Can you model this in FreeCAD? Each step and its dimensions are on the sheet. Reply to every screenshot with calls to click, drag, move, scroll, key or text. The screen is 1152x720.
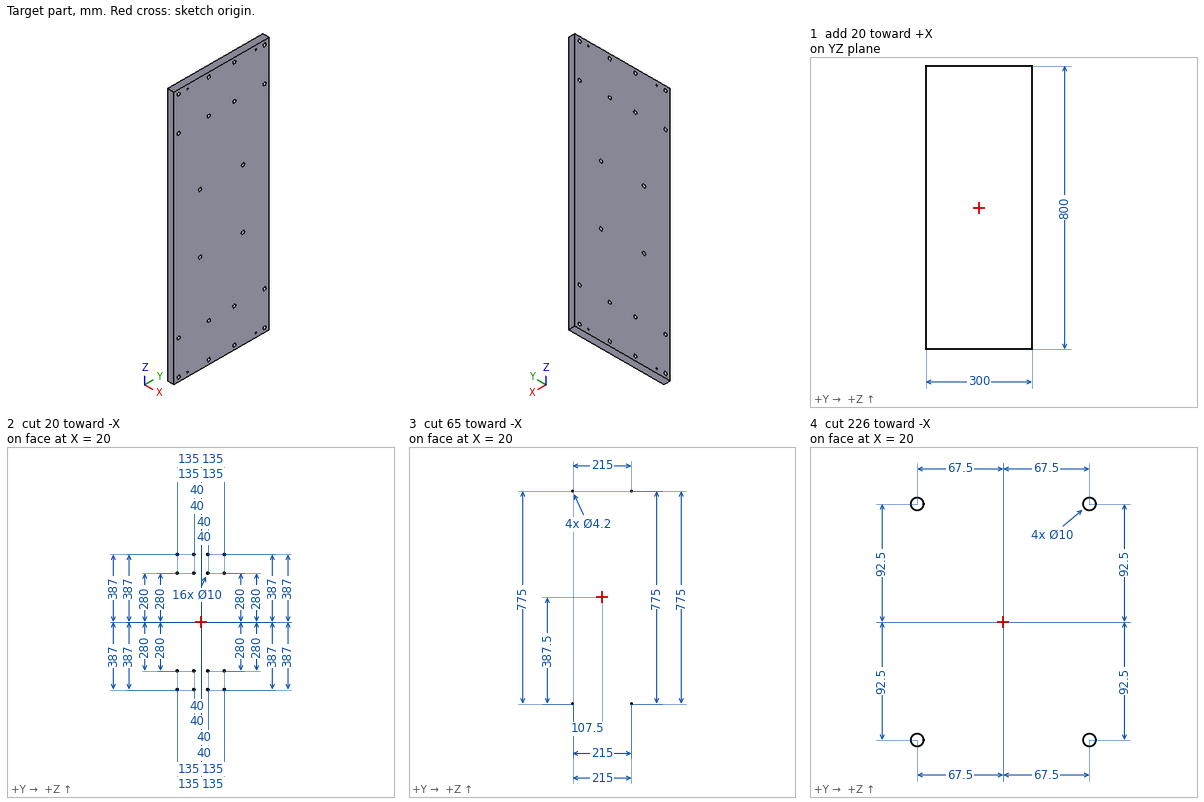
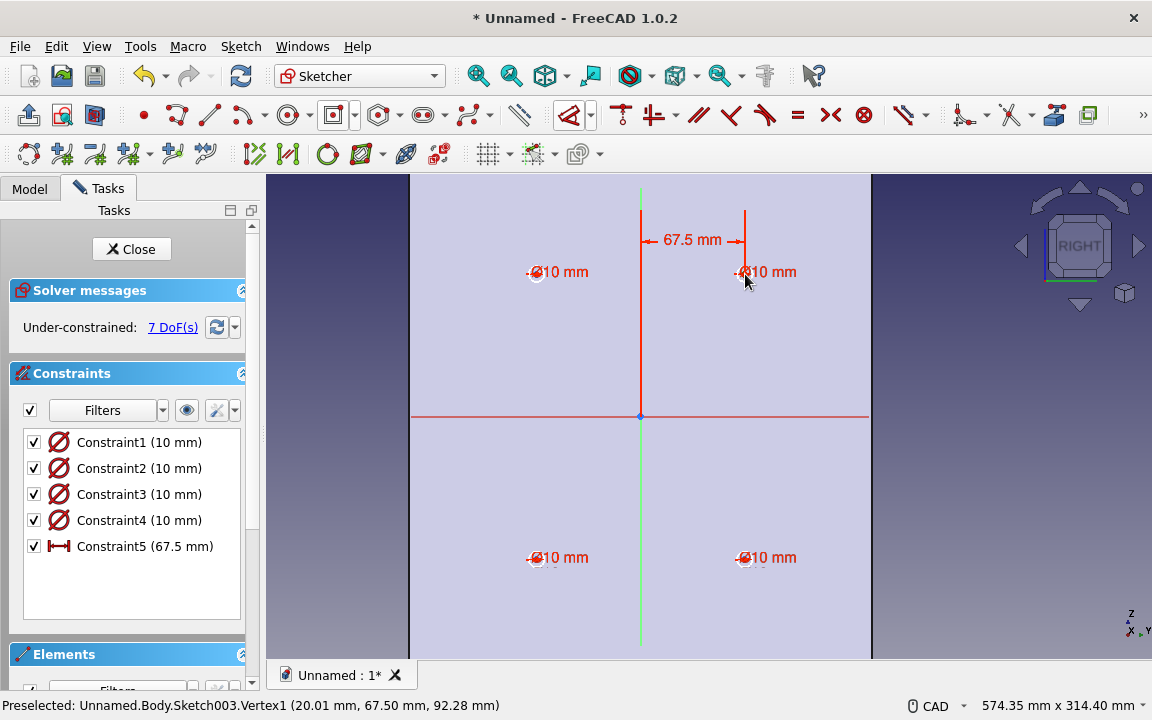
click(590, 116)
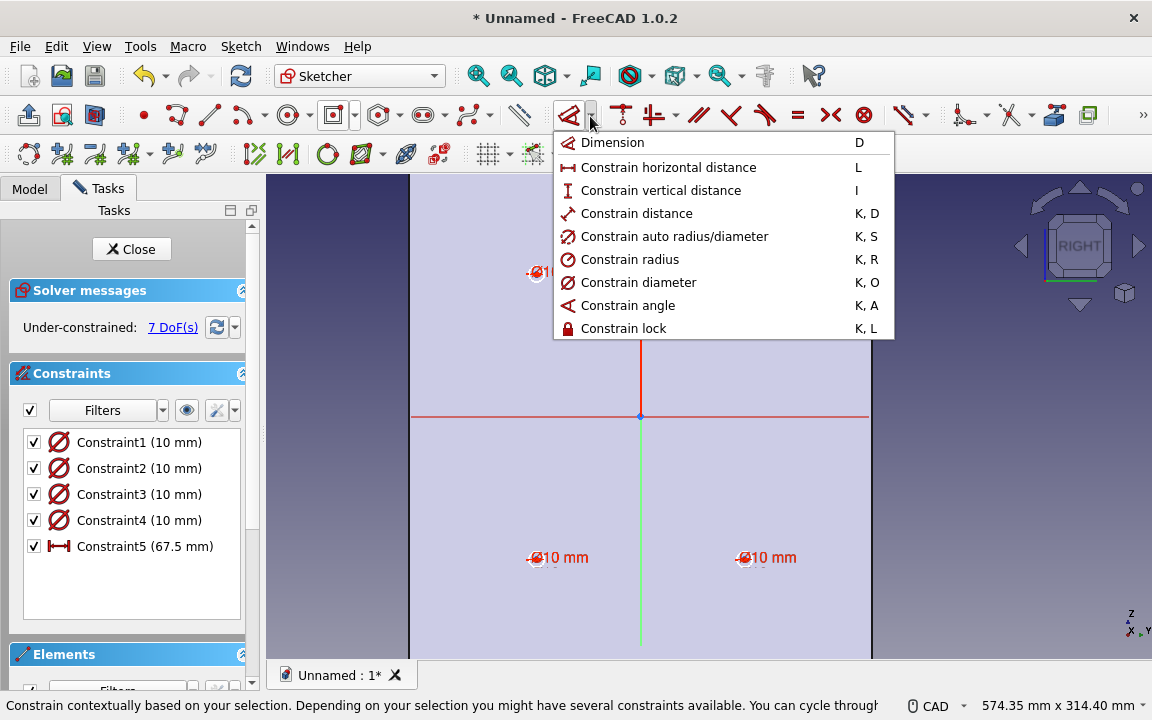
click(724, 190)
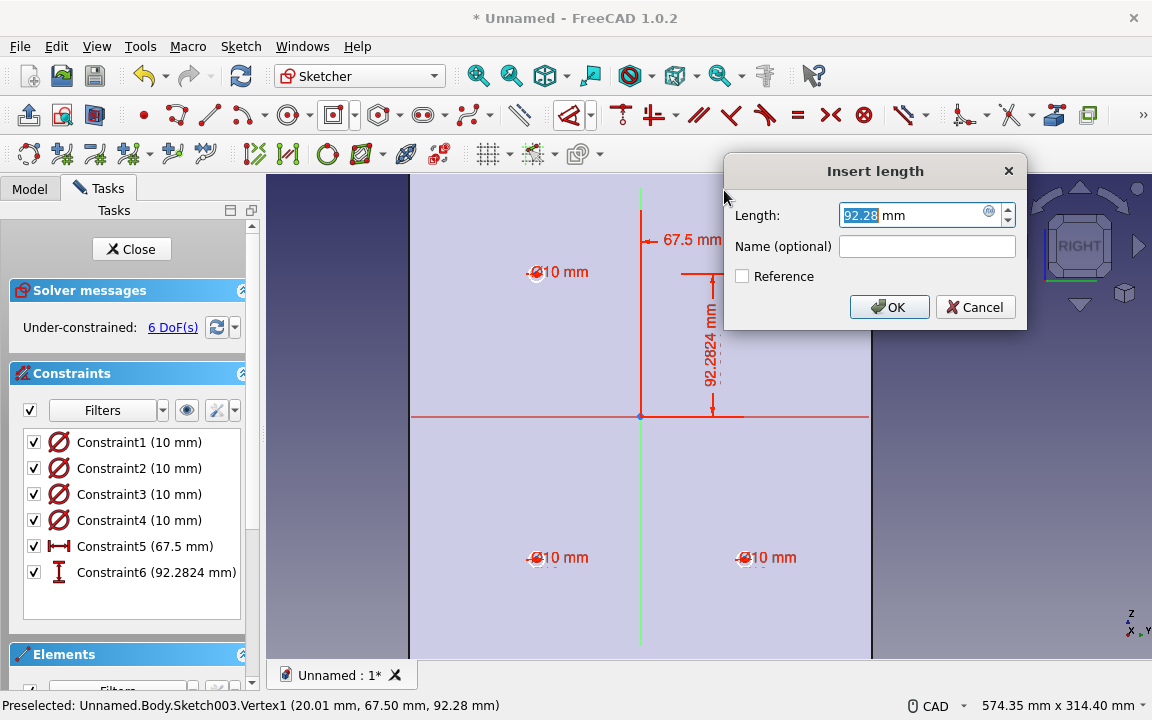
text(92.5)
key(Return)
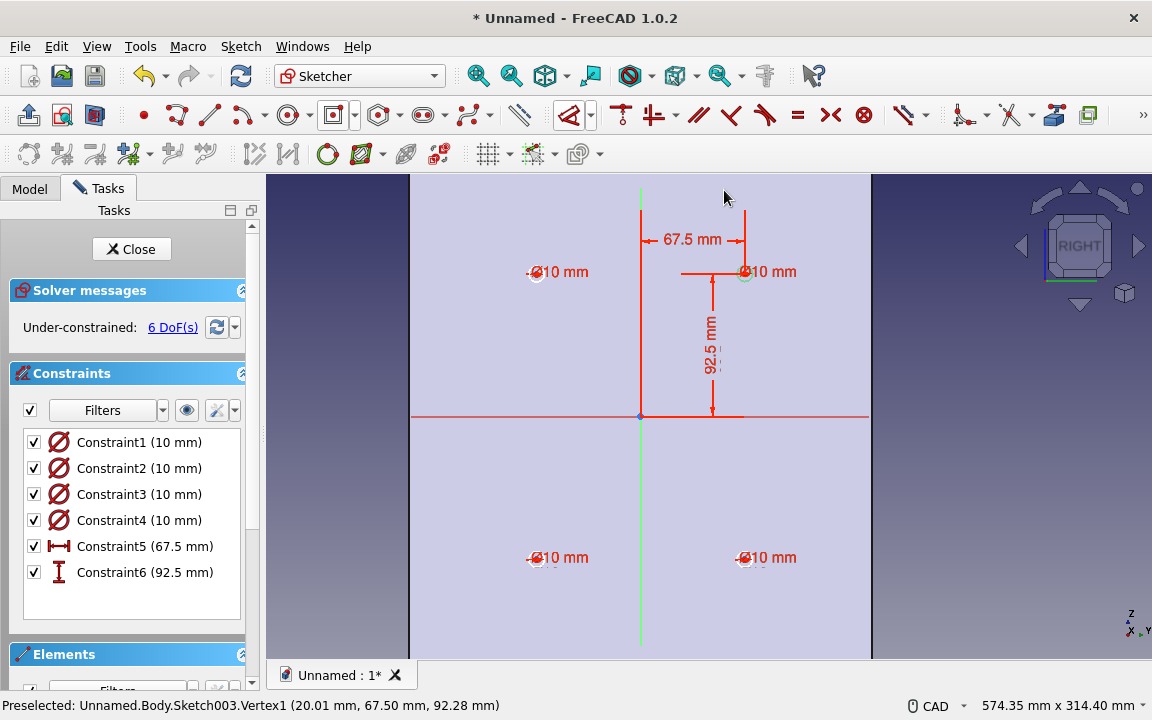
click(745, 560)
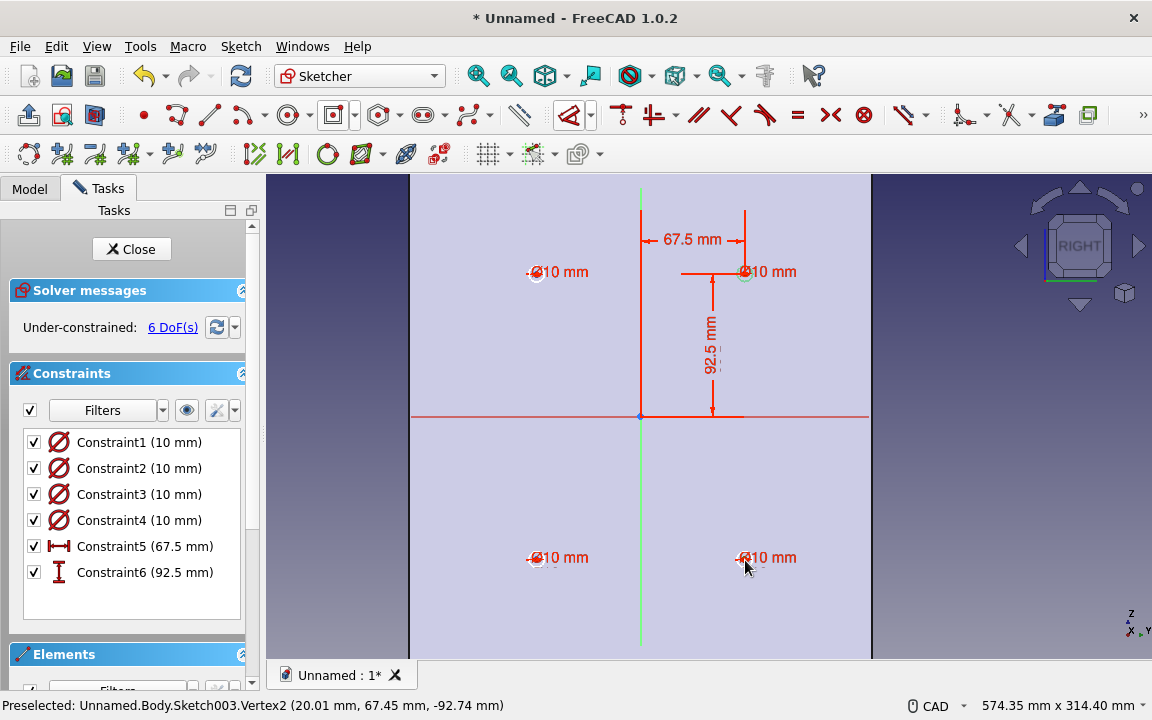
key(l)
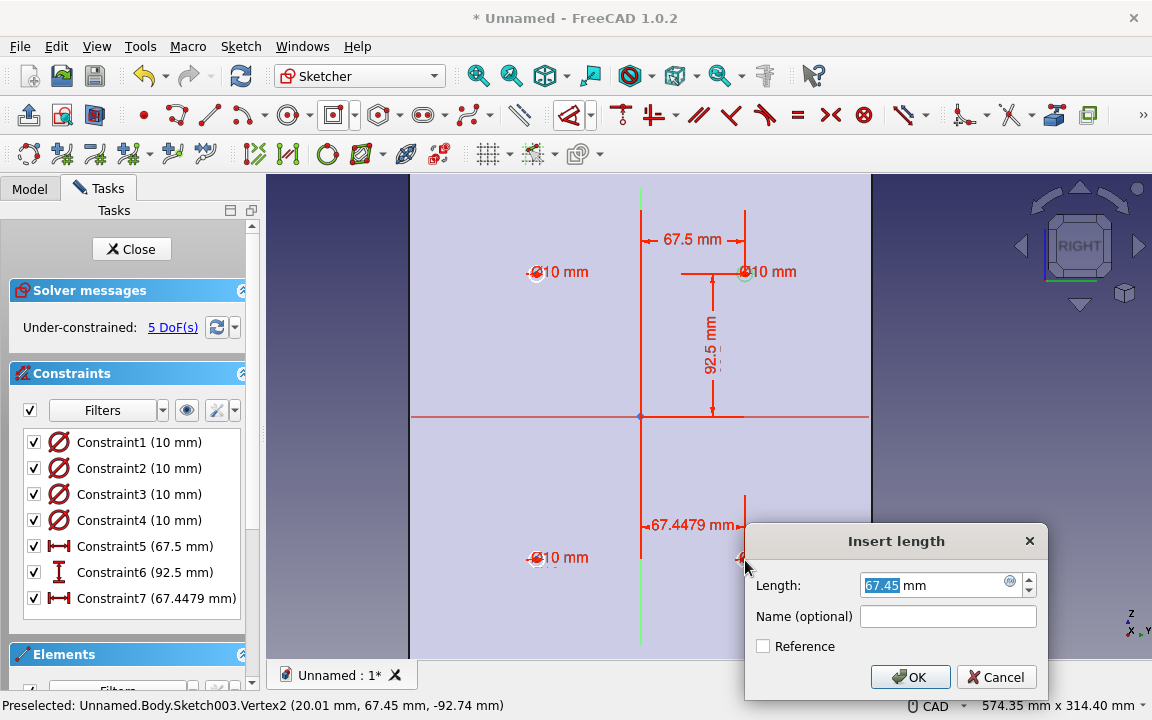
text(67.5)
key(Return)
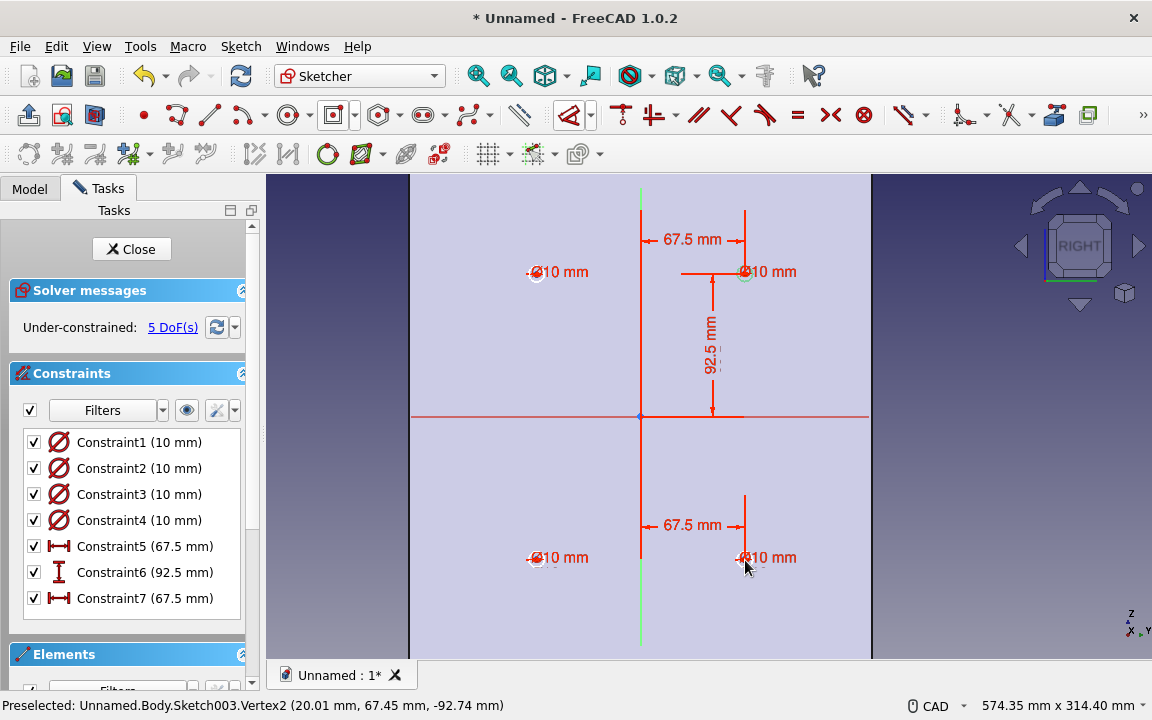
click(745, 560)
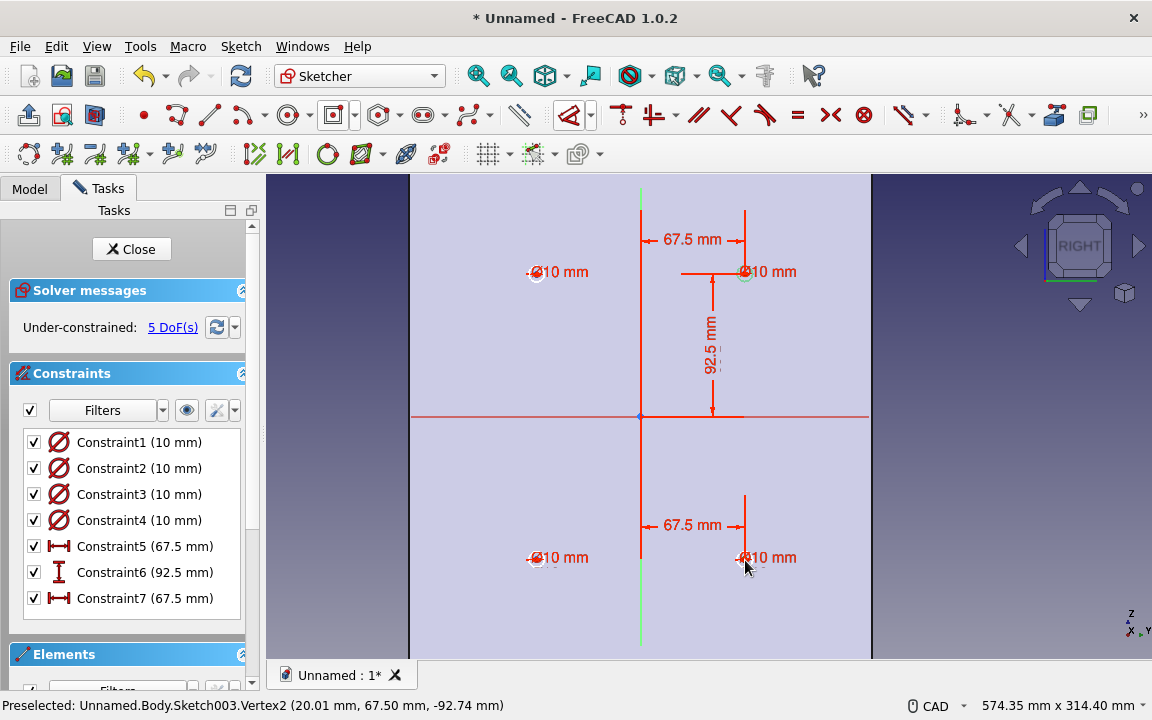
key(i)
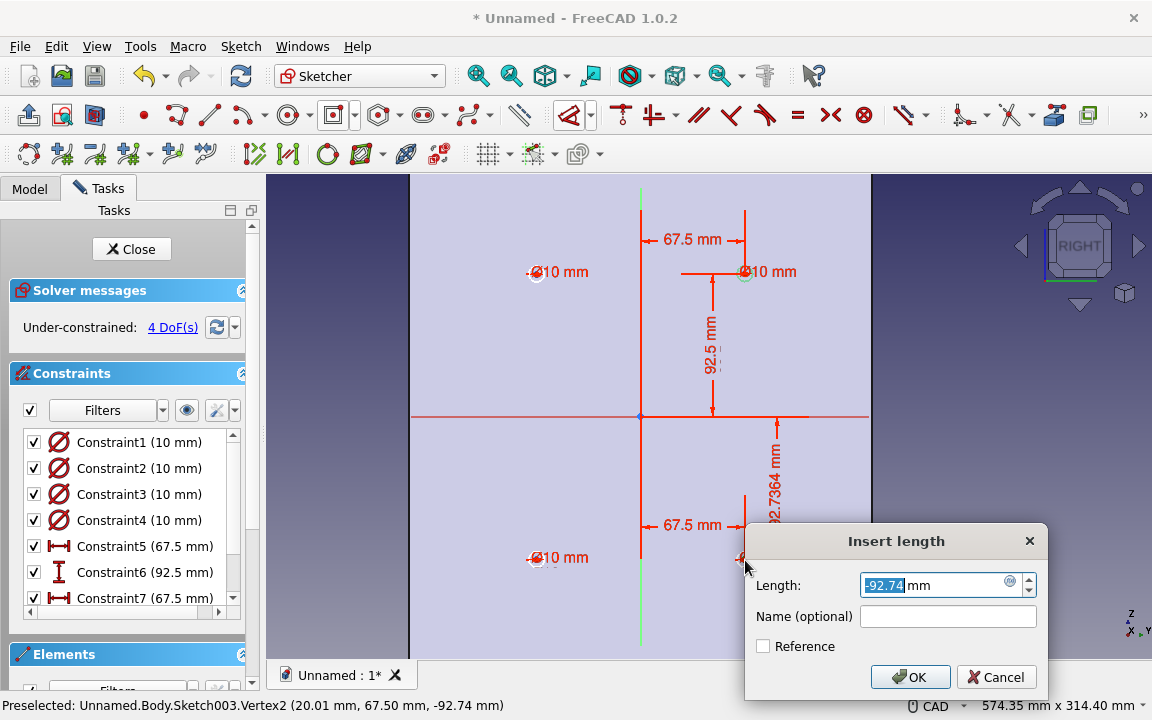
text(-92.5)
key(Return)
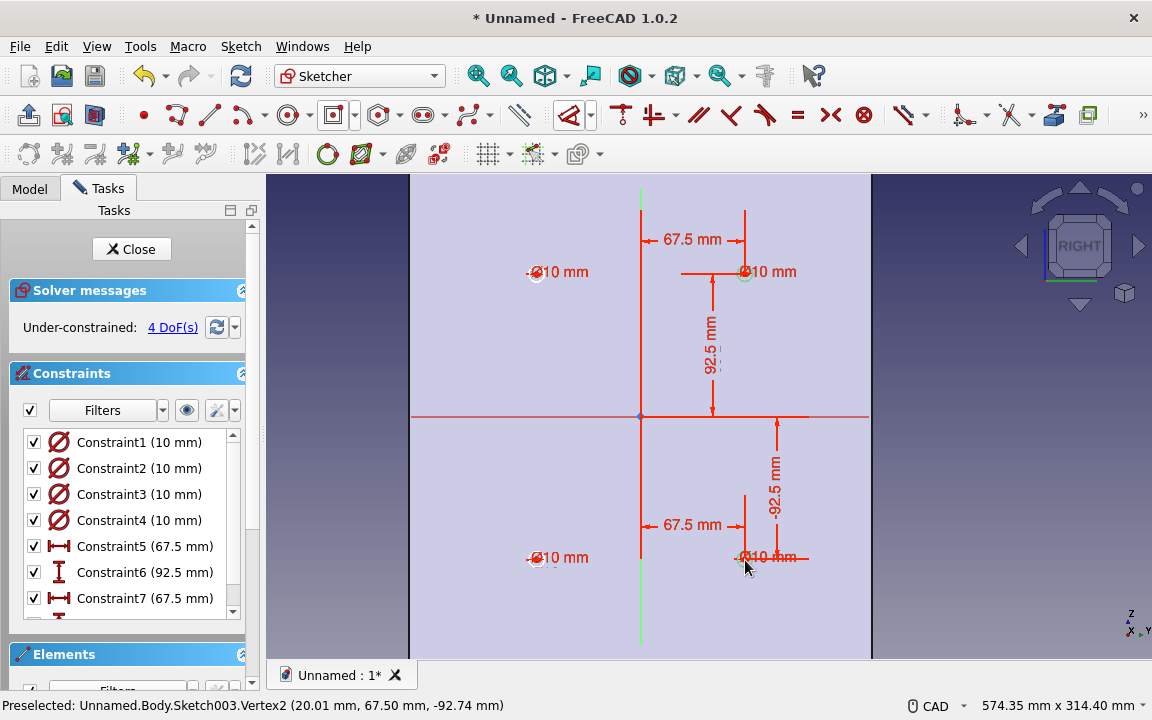
click(537, 560)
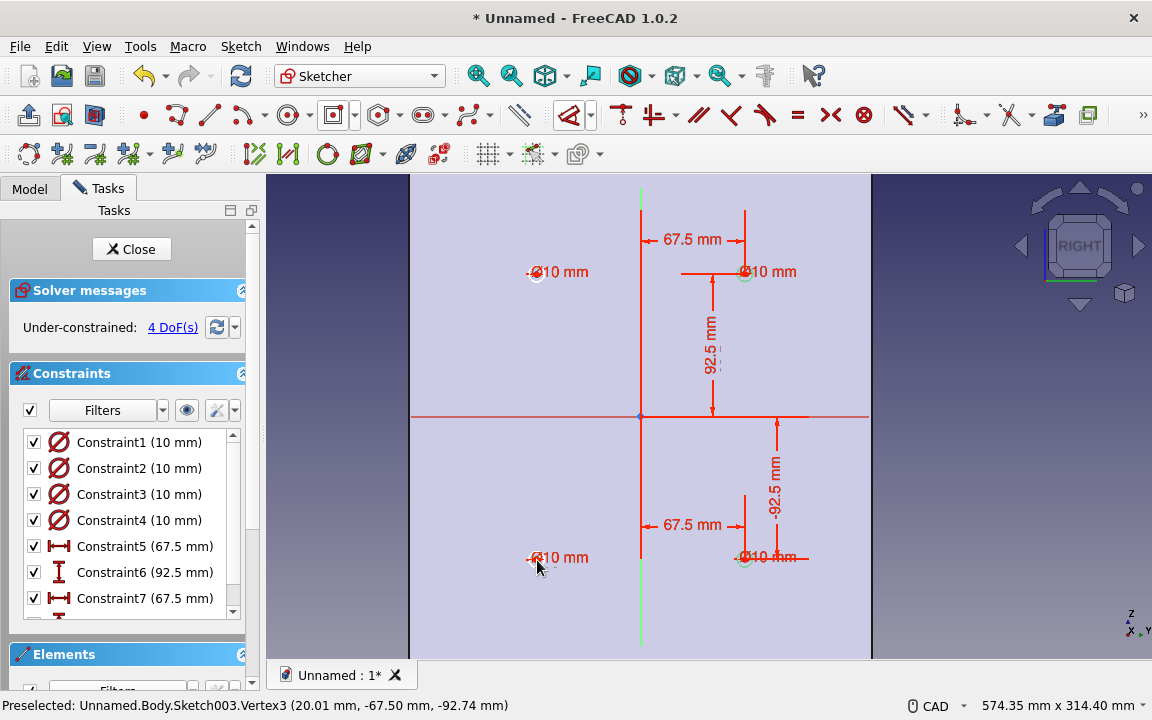
key(l)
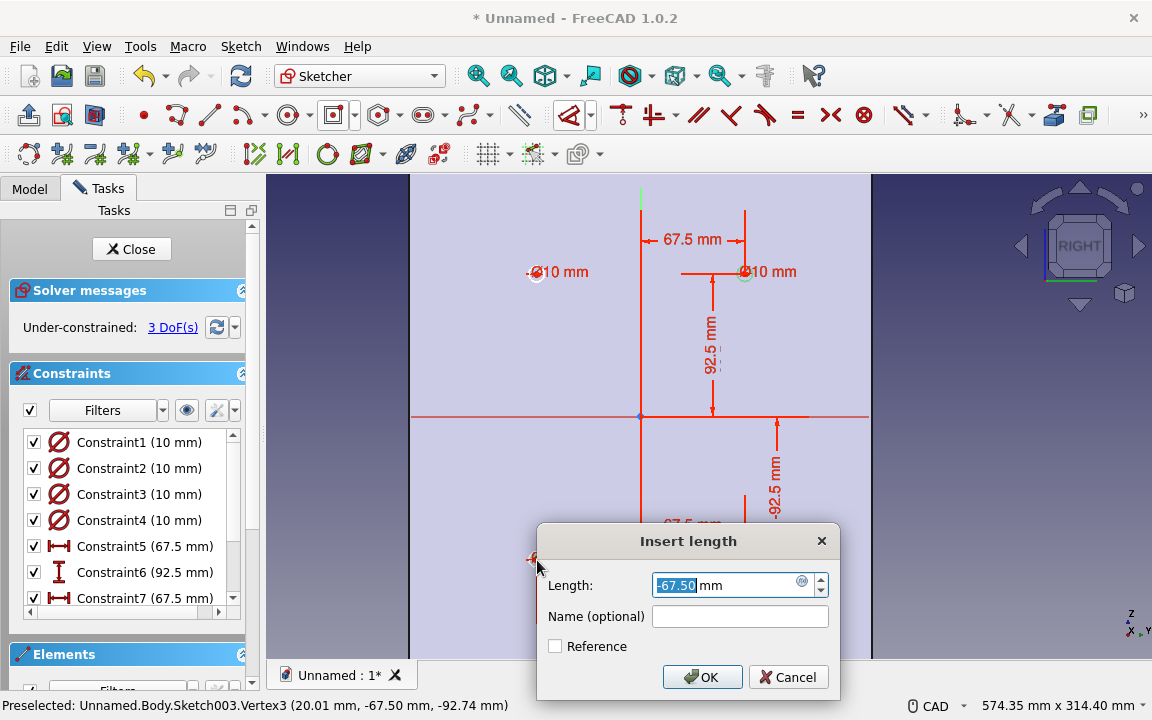
text(-67.5)
key(Return)